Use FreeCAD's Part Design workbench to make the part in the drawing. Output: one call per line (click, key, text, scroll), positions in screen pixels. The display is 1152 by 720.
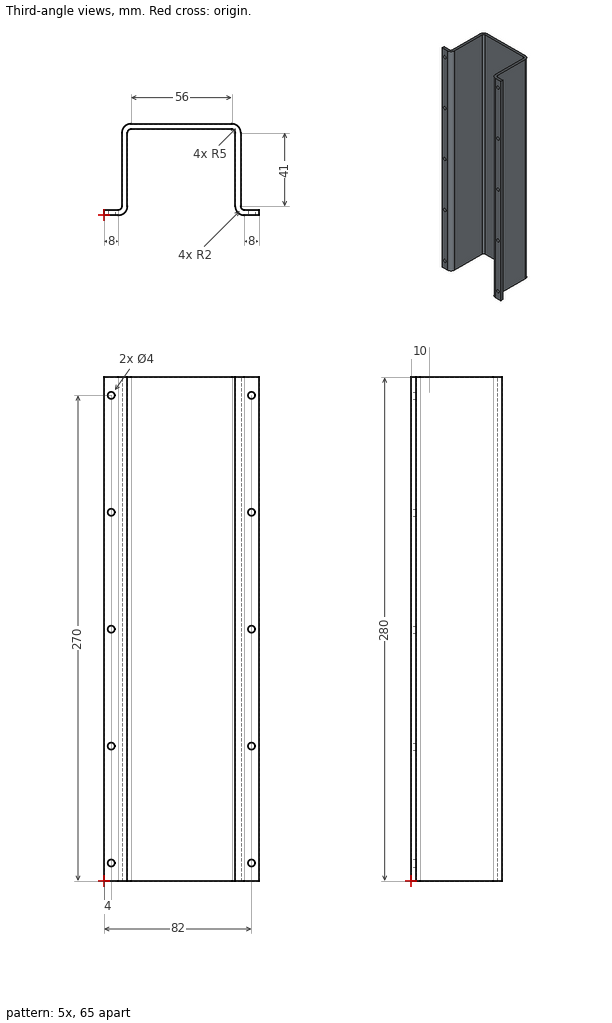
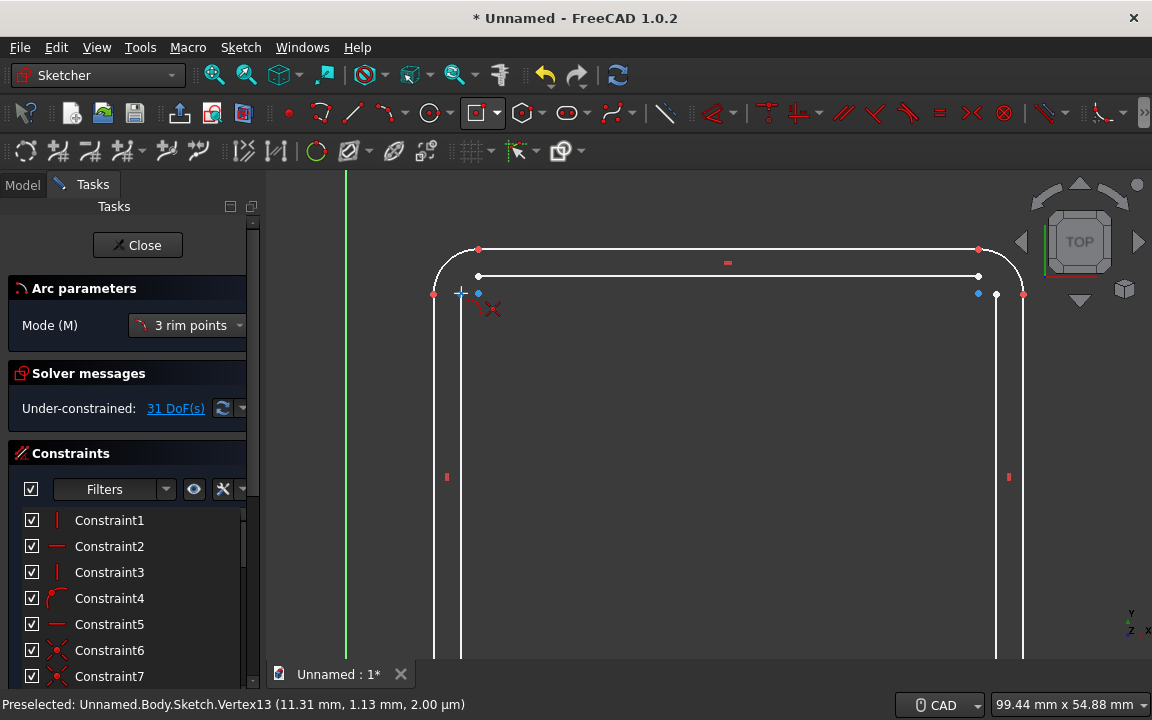
click(461, 294)
click(479, 276)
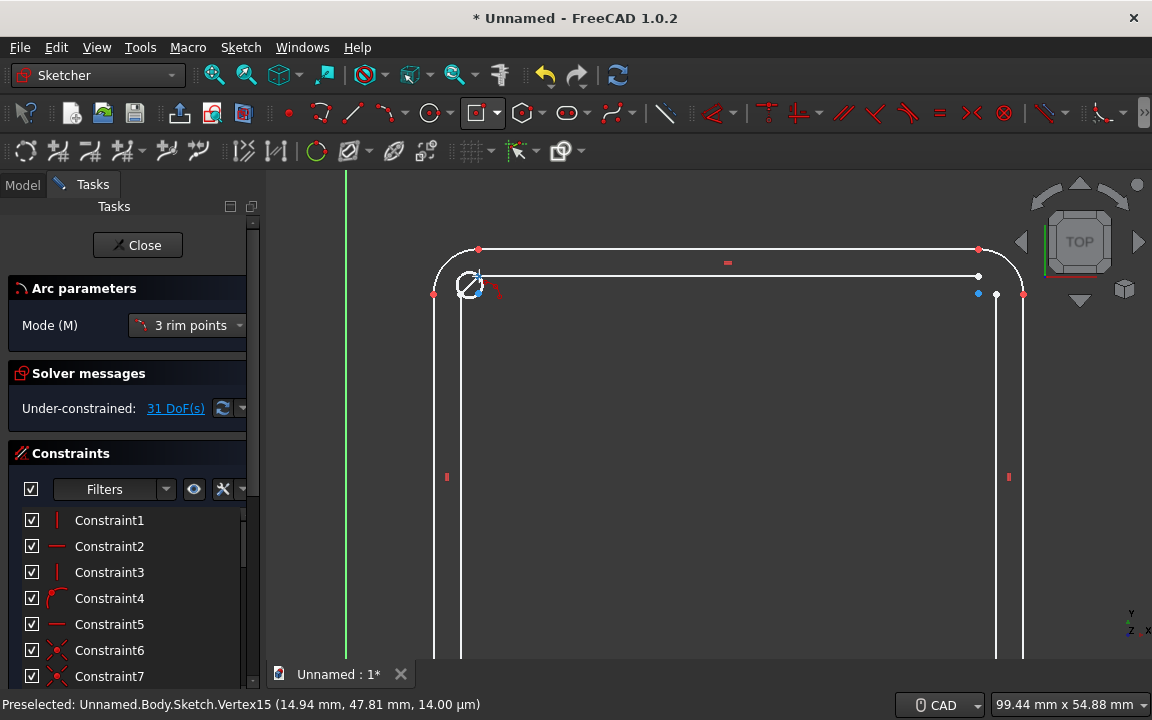
scroll(467, 280, up, 6)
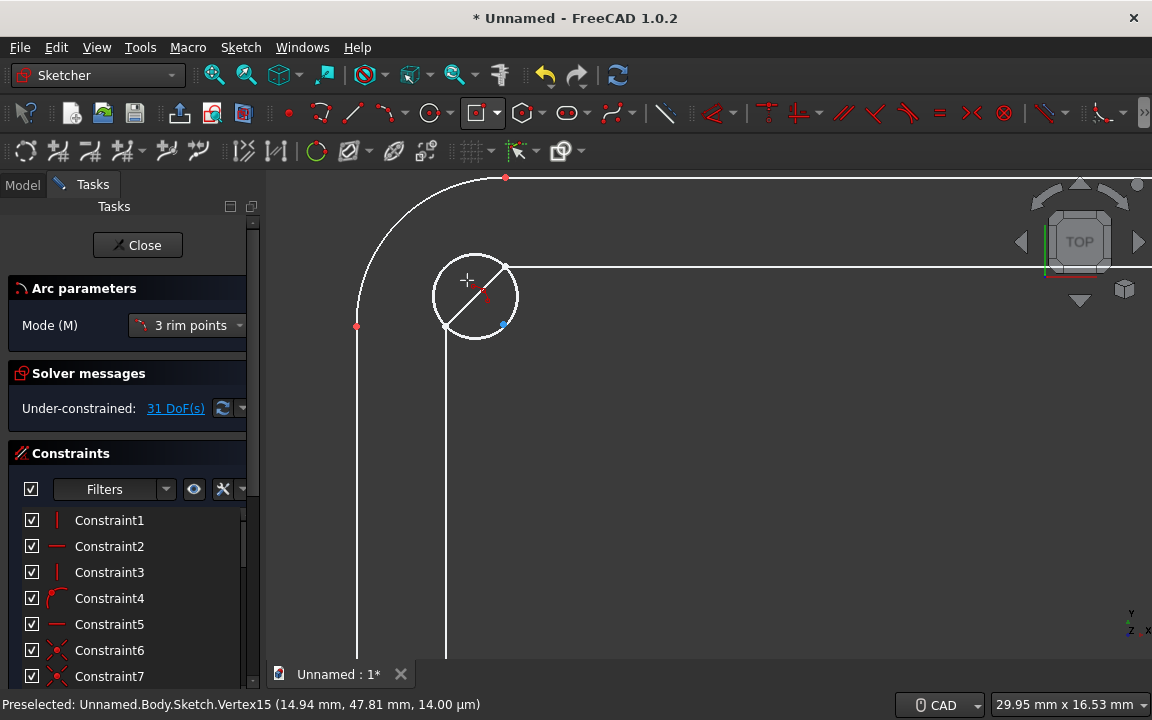
click(465, 278)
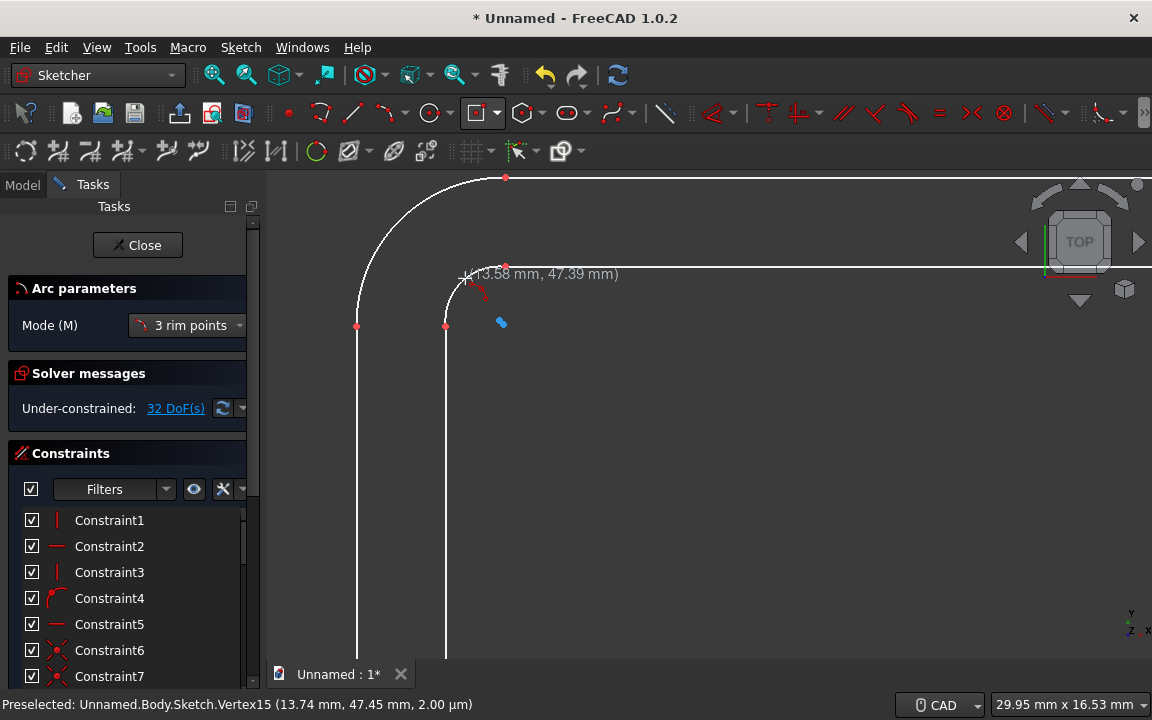
scroll(465, 285, down, 8)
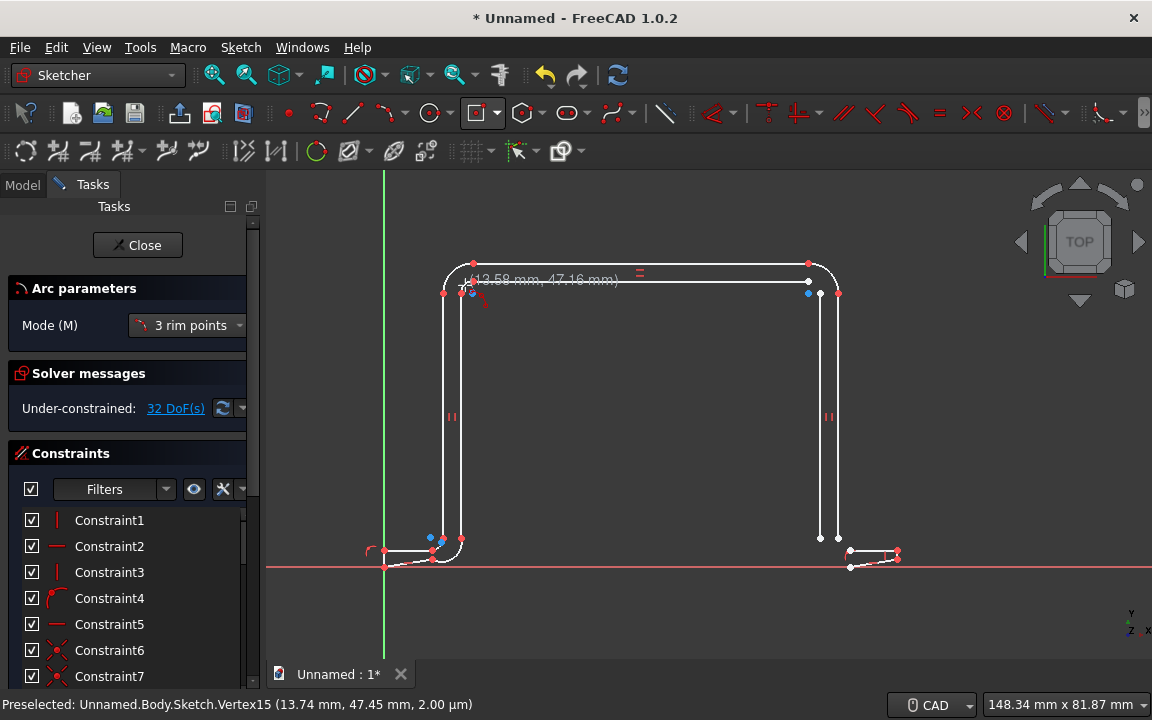
scroll(808, 280, up, 2)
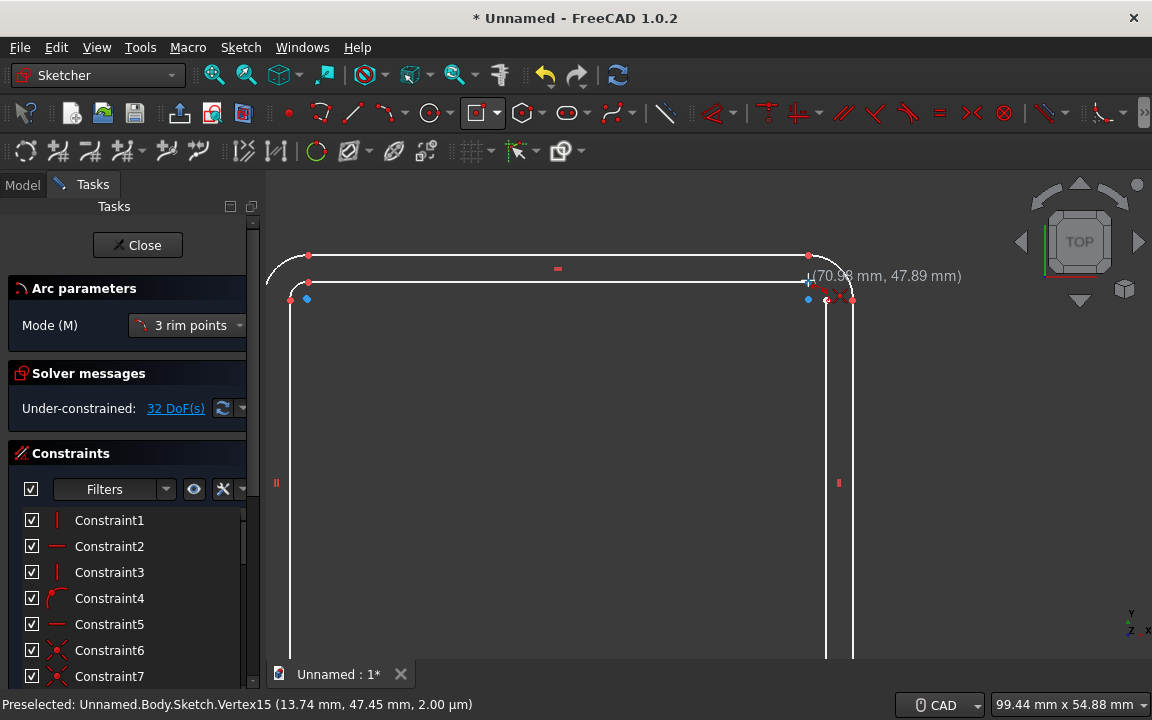
click(808, 282)
click(826, 300)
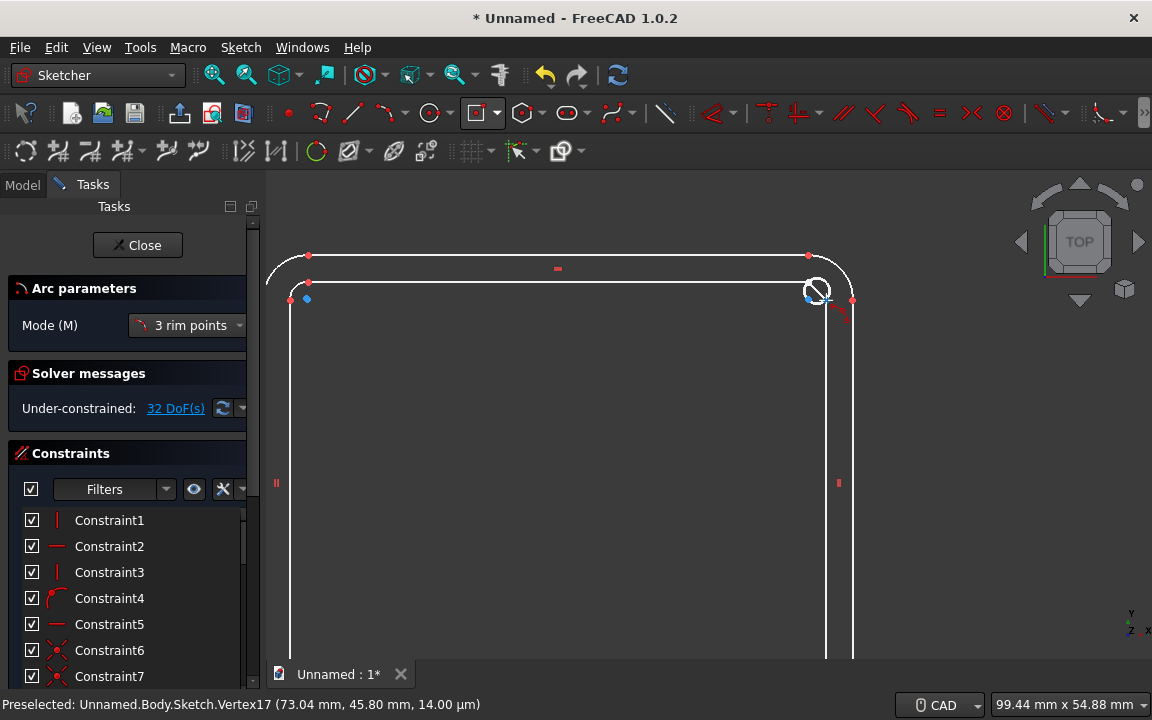
scroll(820, 286, up, 6)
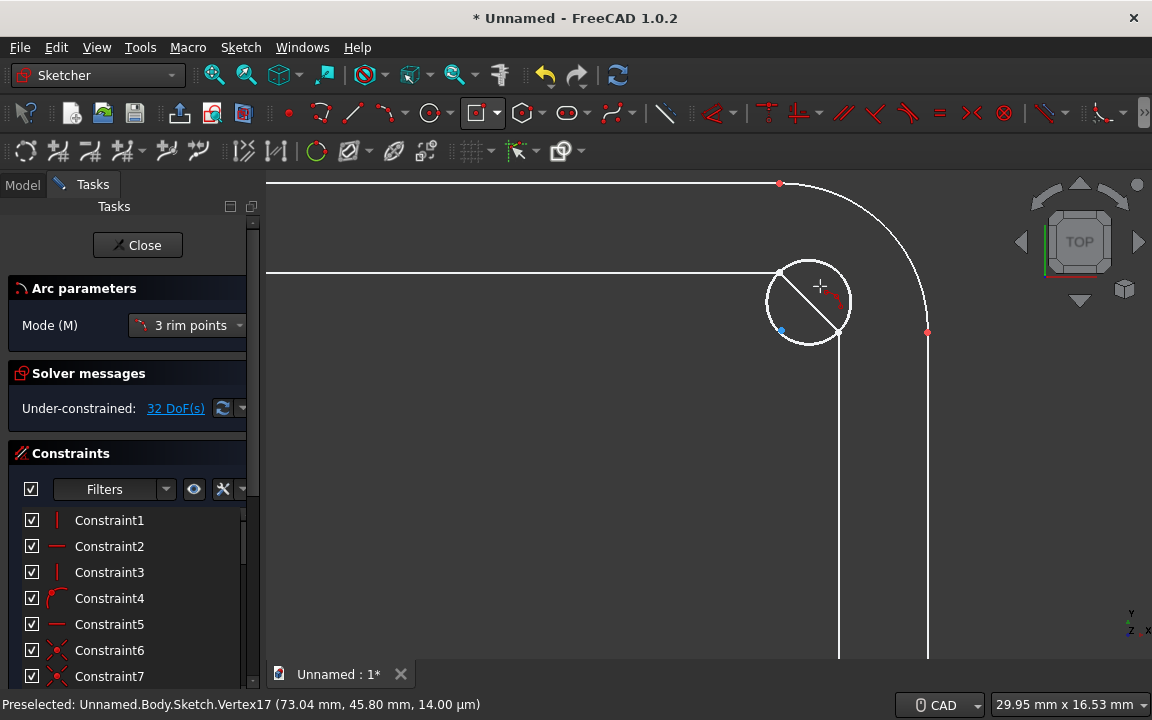
click(820, 284)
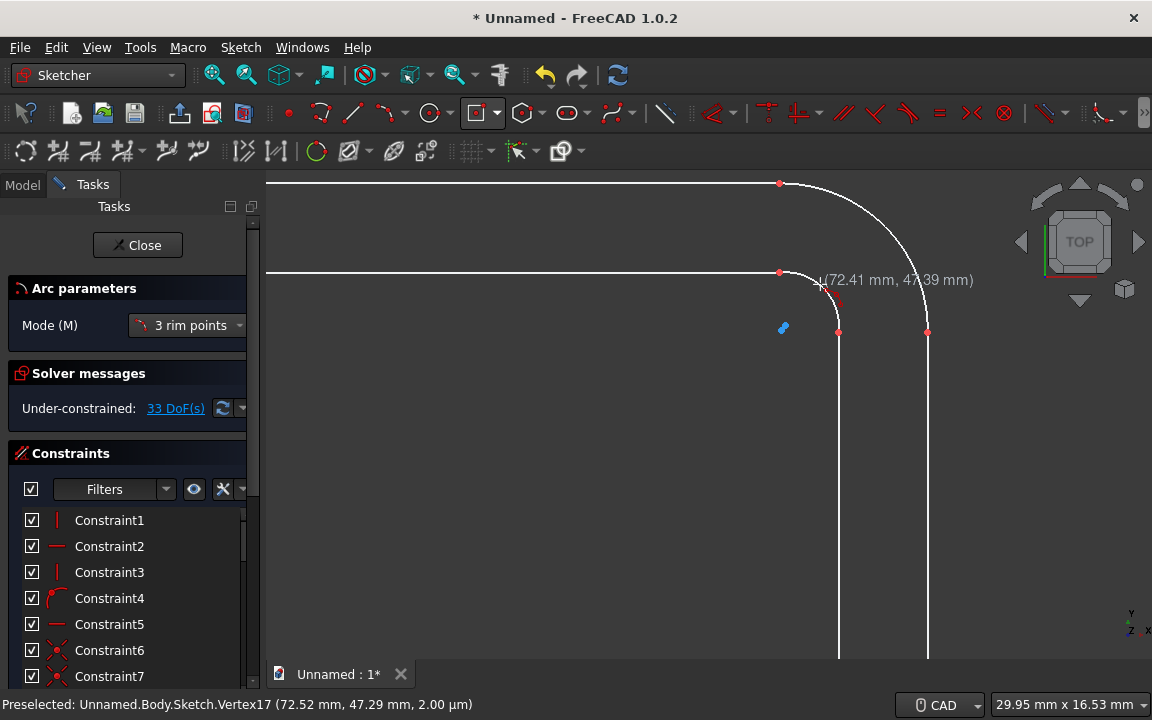
scroll(815, 283, down, 8)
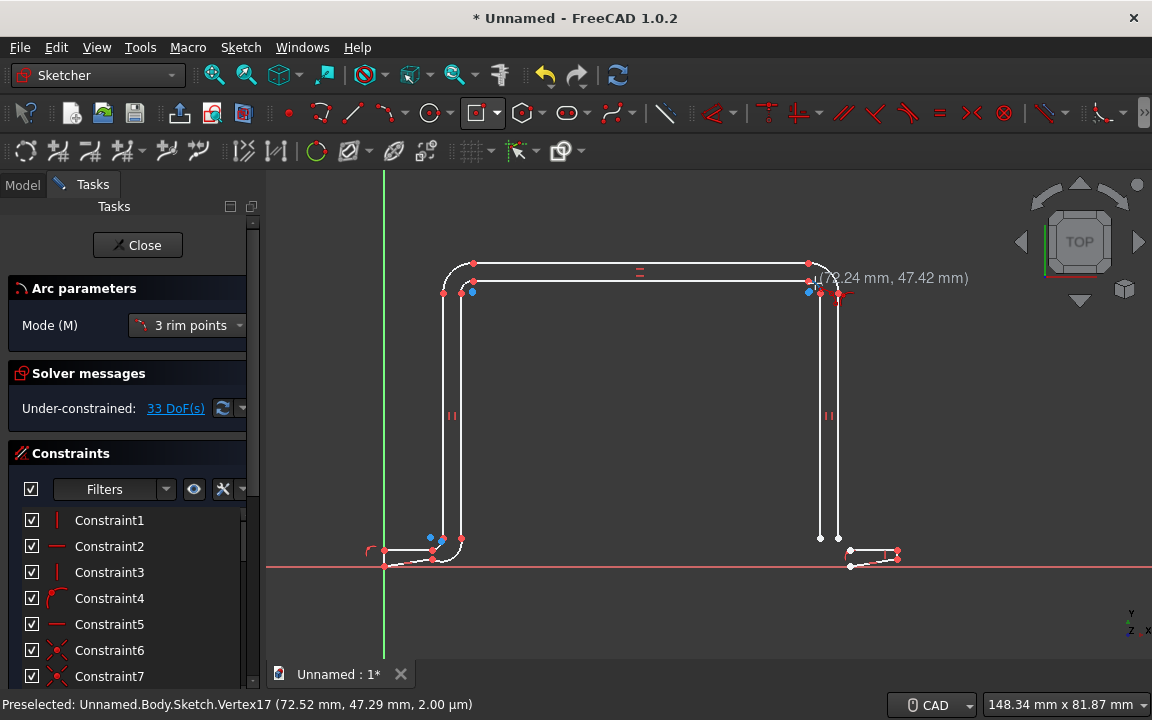
click(820, 538)
click(850, 567)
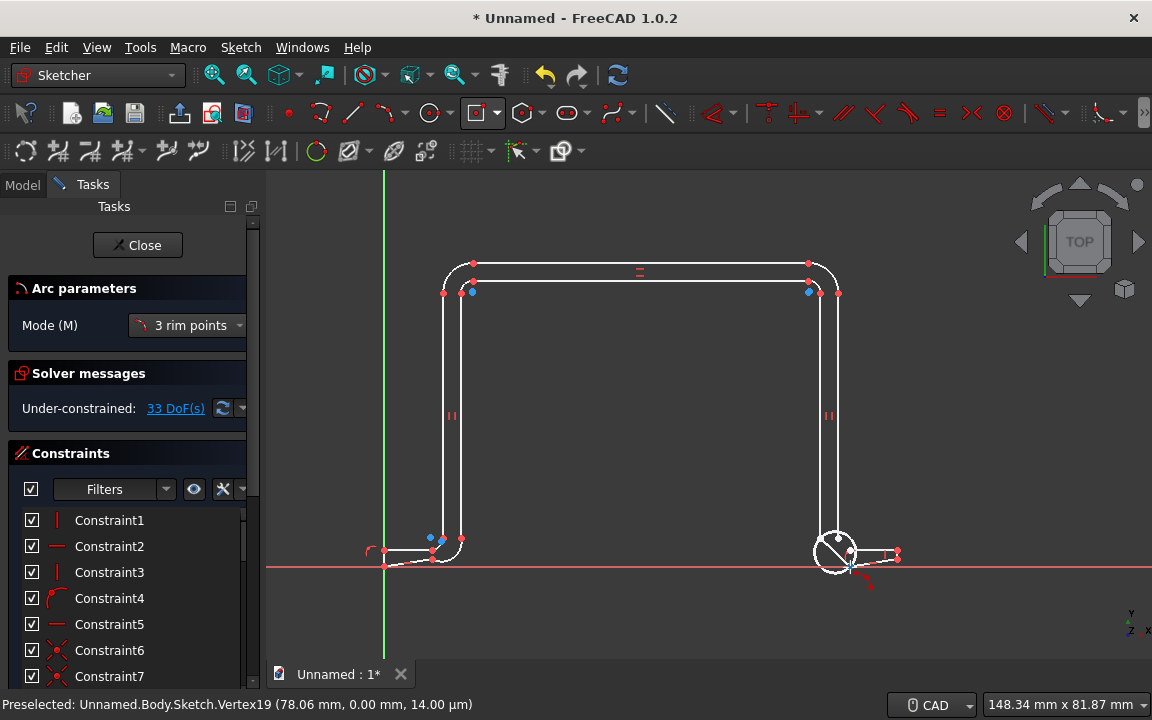
scroll(829, 558, up, 3)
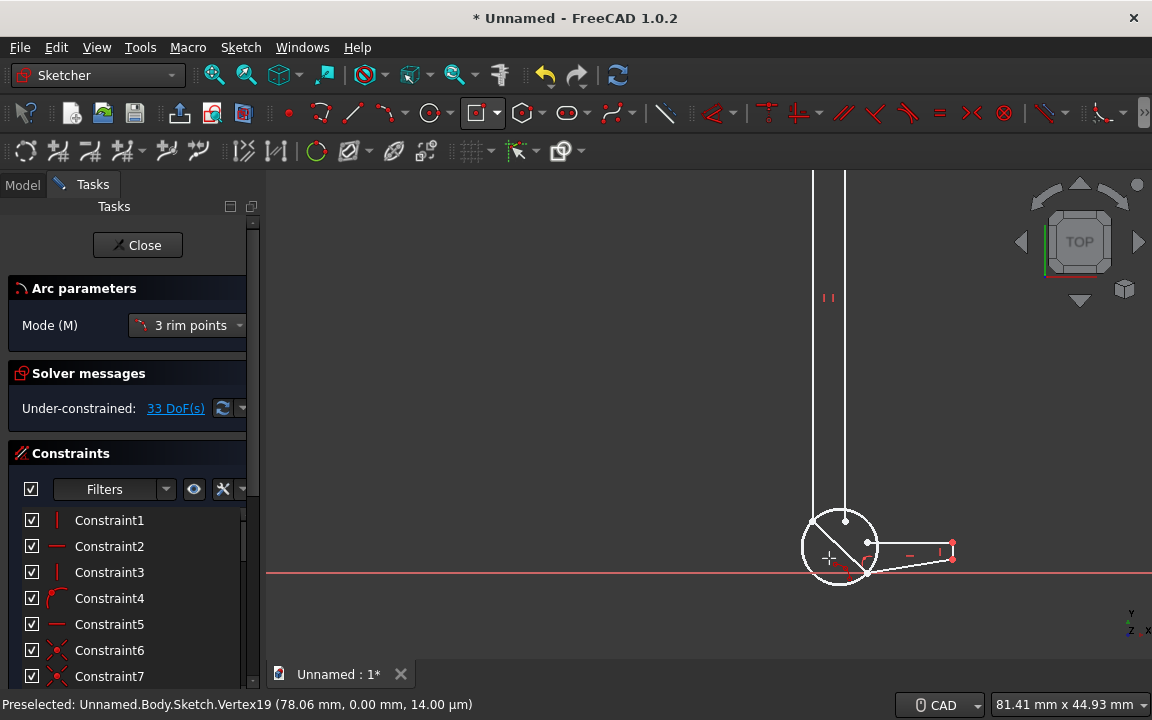
click(828, 557)